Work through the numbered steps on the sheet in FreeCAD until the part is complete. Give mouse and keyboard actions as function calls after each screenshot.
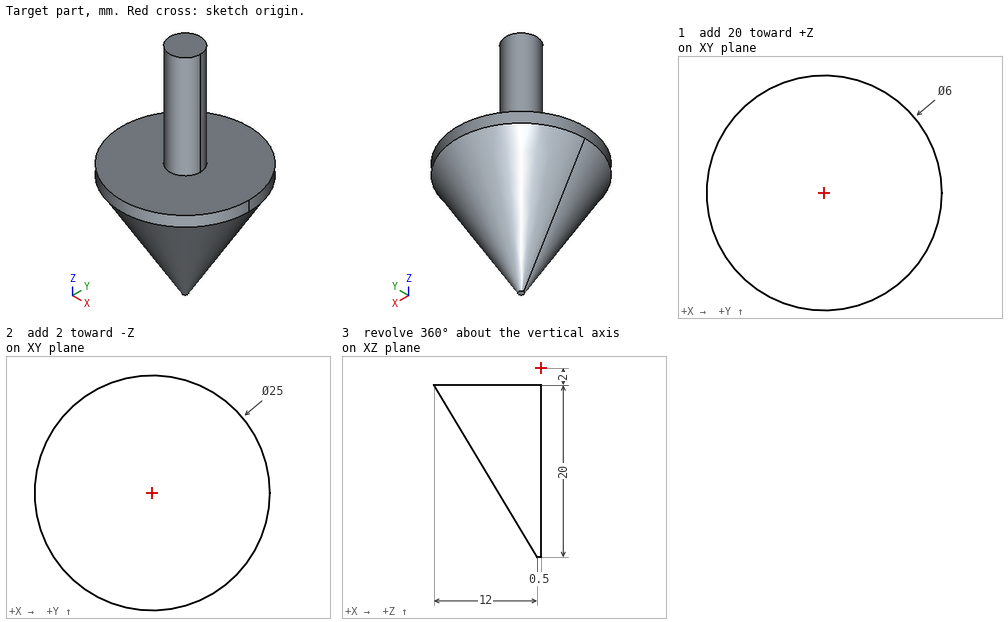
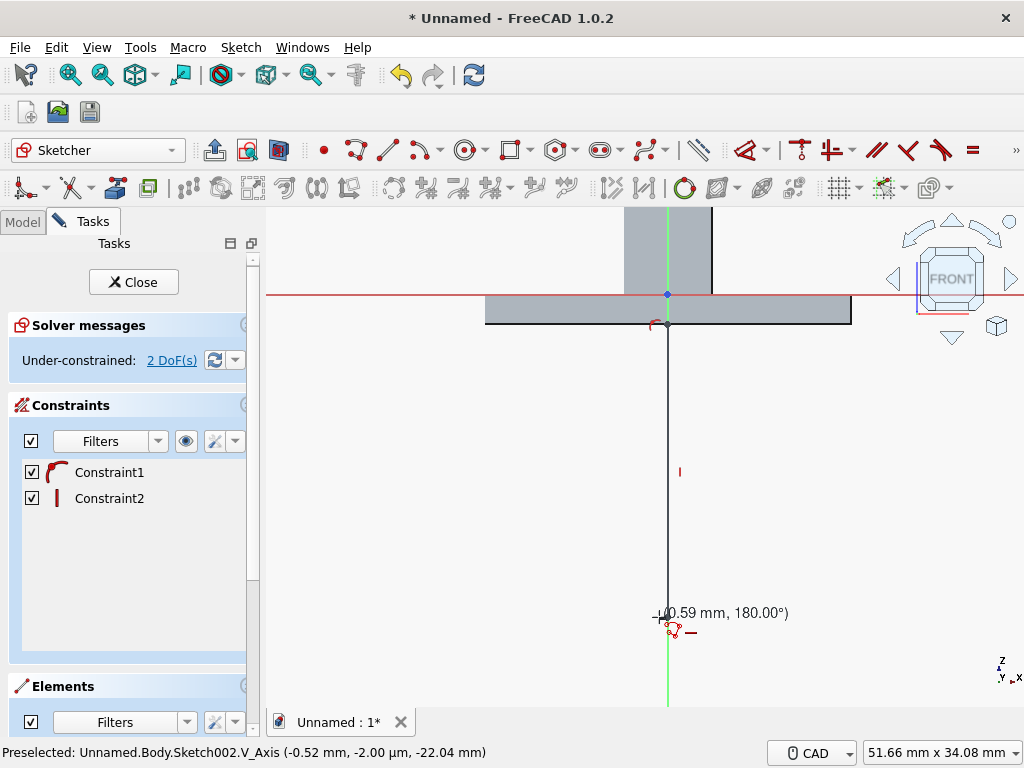
scroll(660, 617, up, 4)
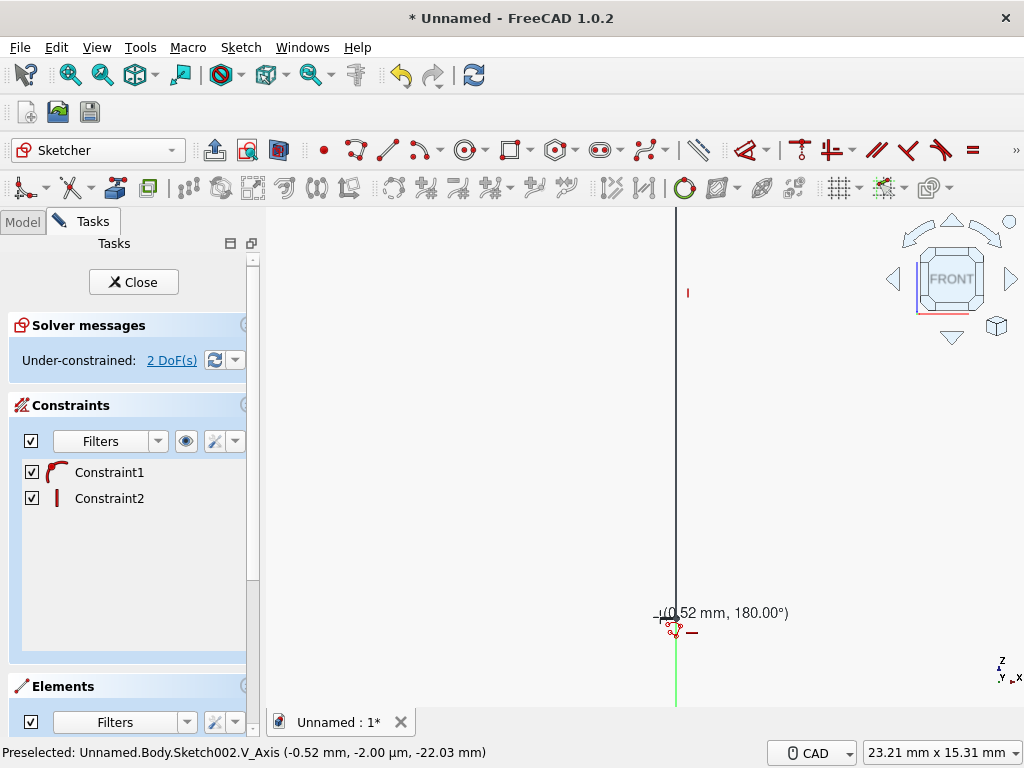
click(660, 616)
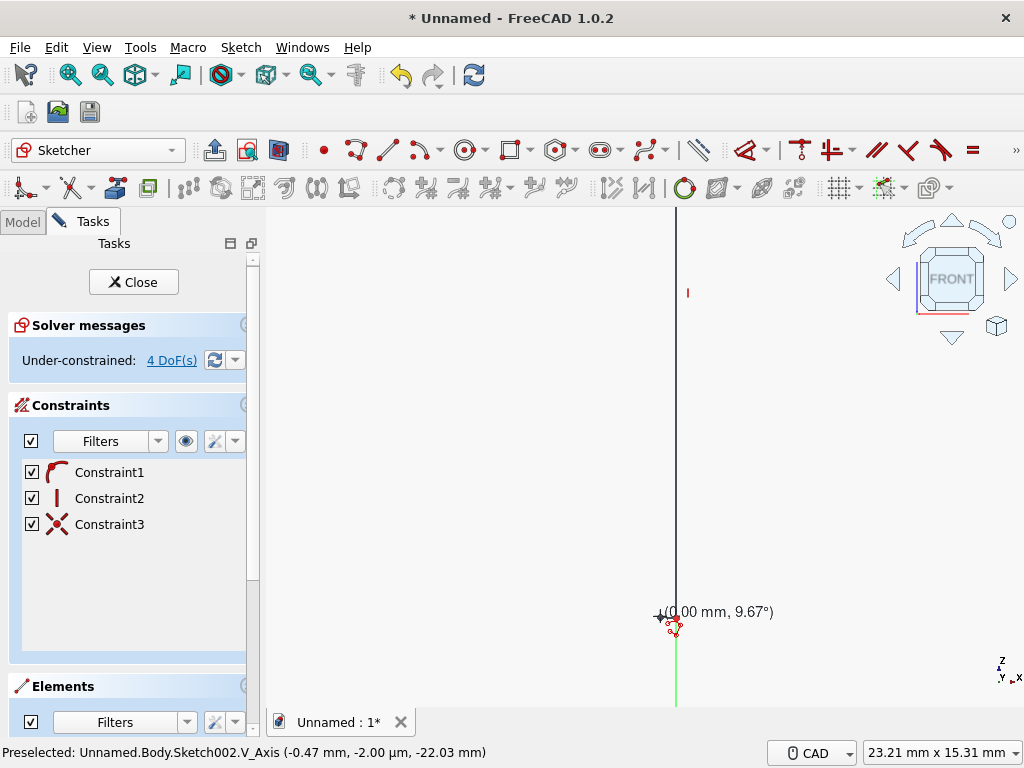
scroll(662, 619, down, 4)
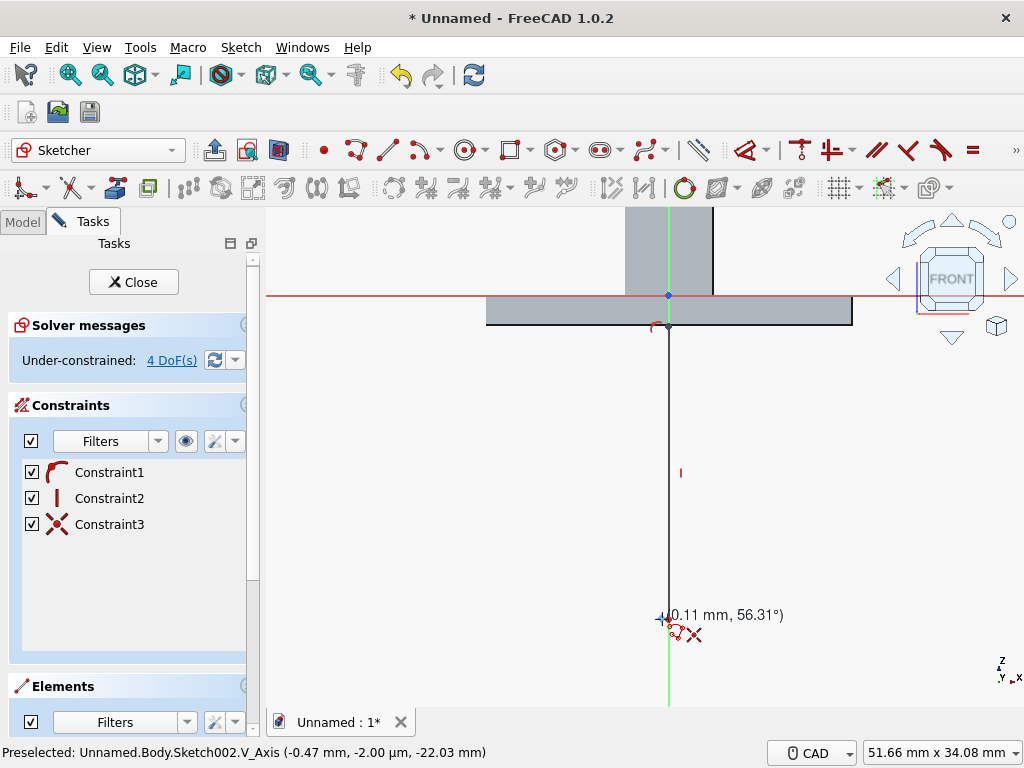
click(485, 325)
click(669, 326)
key(Escape)
key(Escape)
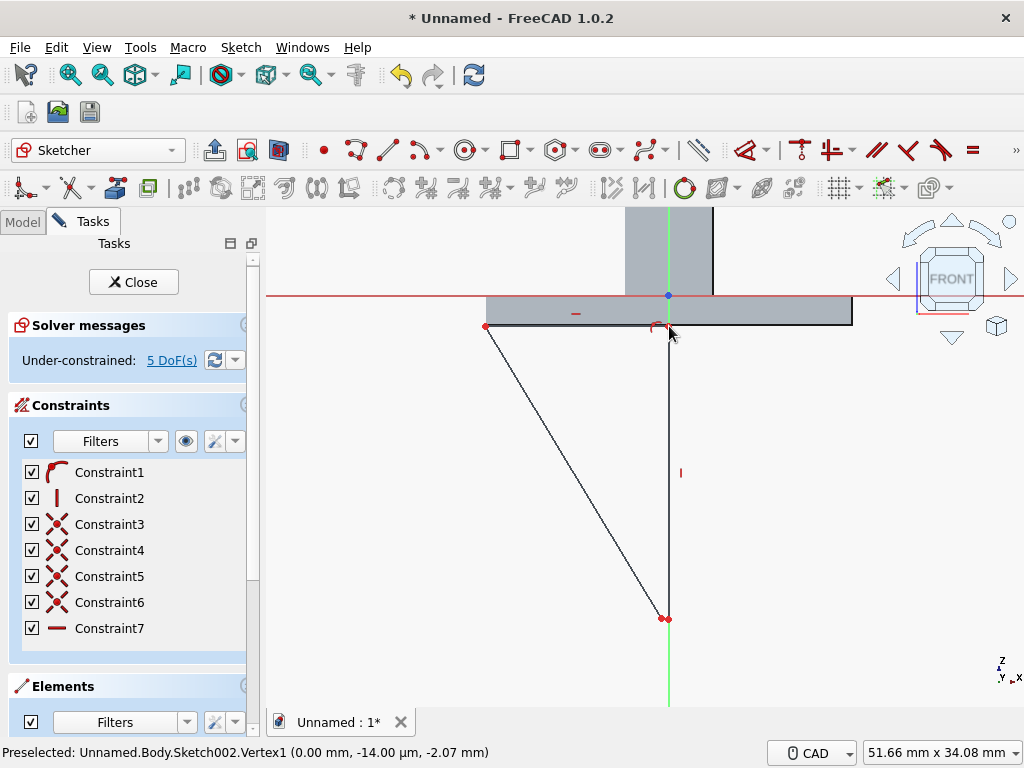
scroll(665, 619, up, 7)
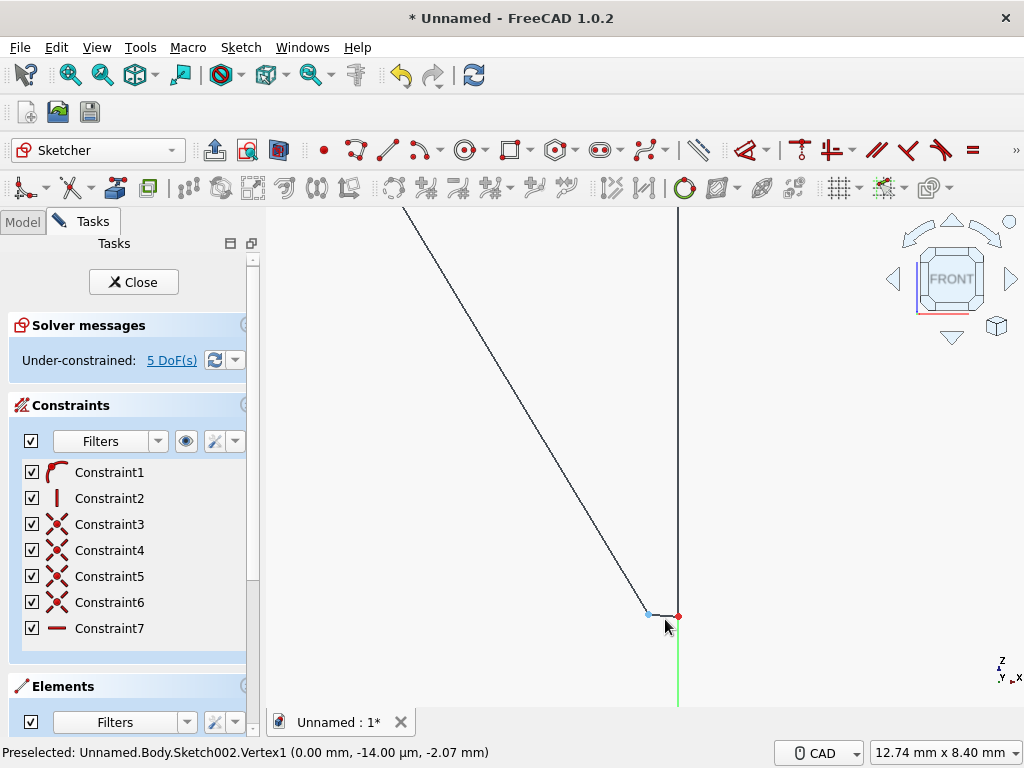
click(664, 616)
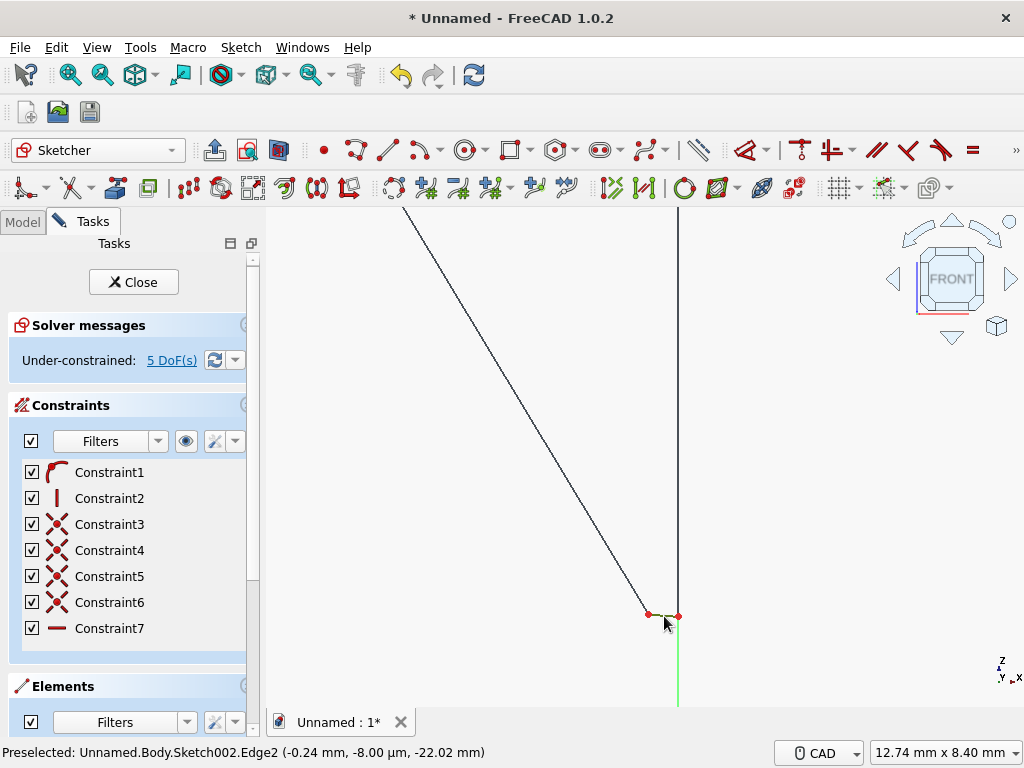
key(h)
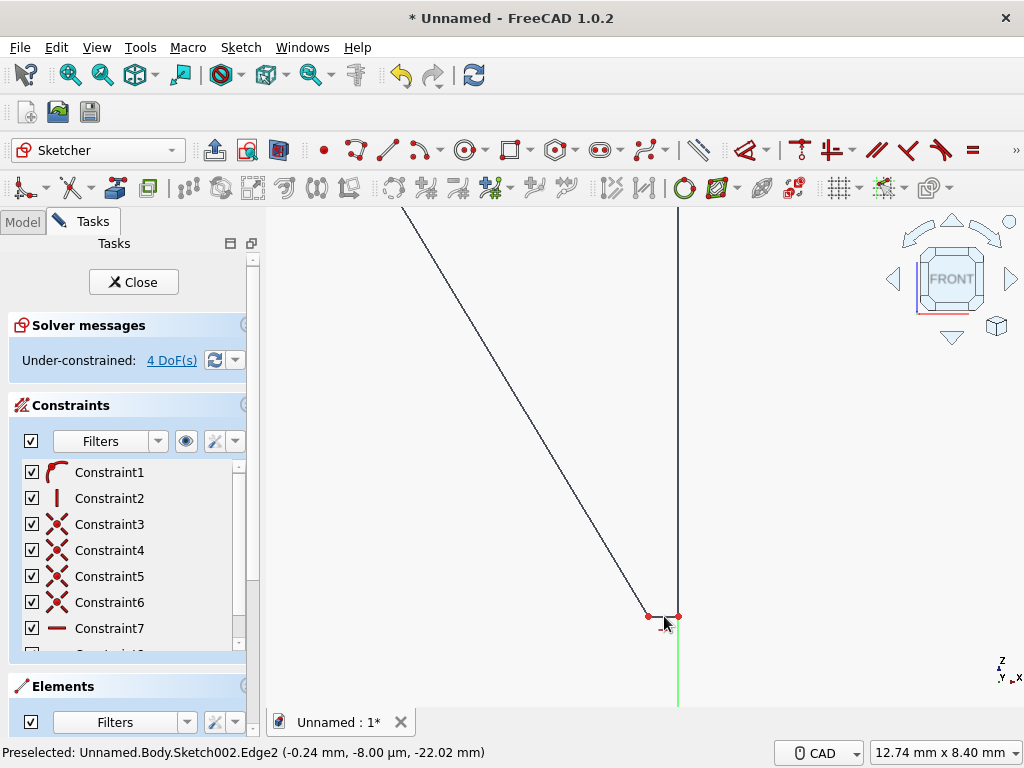
click(746, 150)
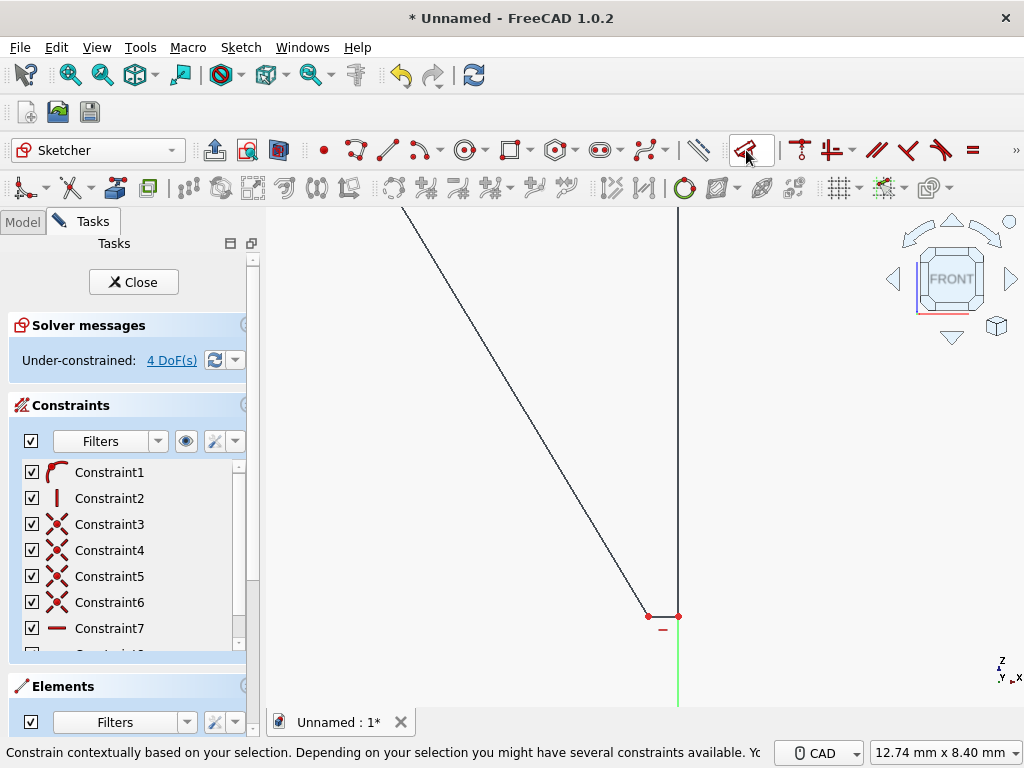
scroll(665, 620, down, 7)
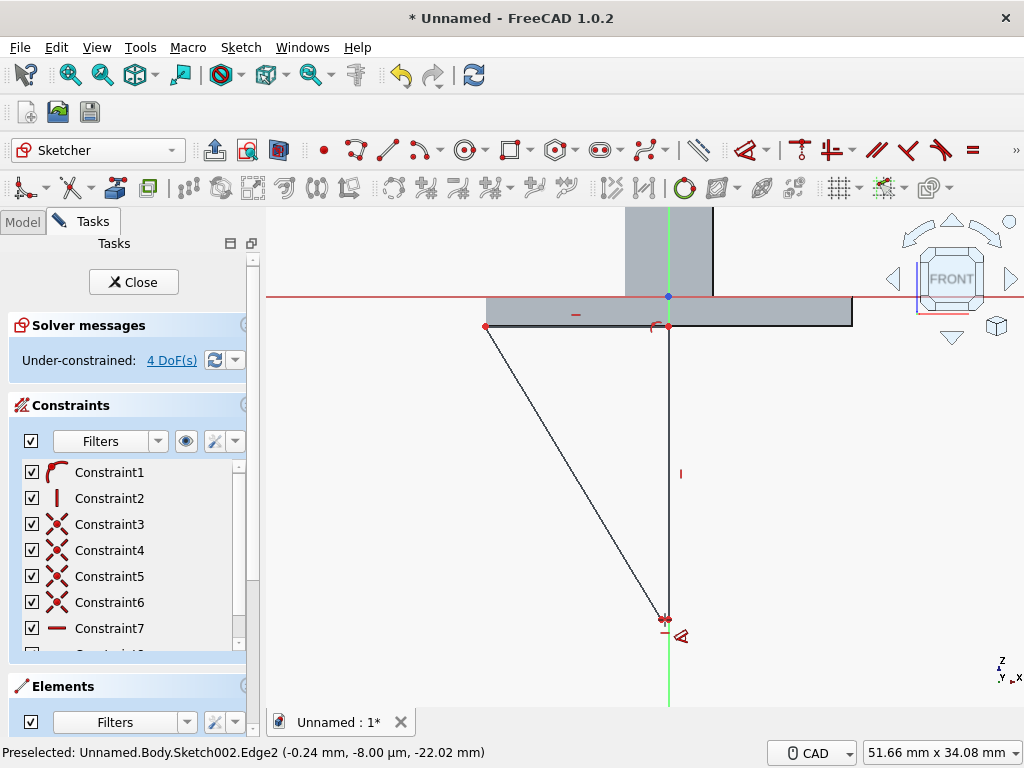
click(669, 532)
click(703, 473)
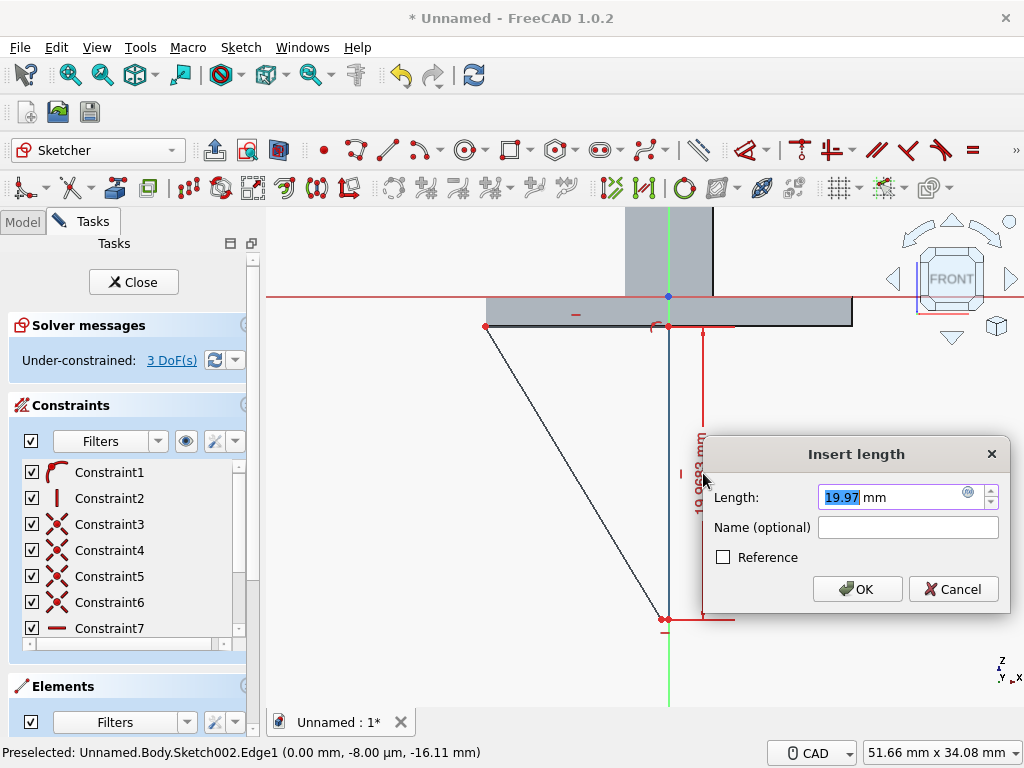
text(20)
key(Return)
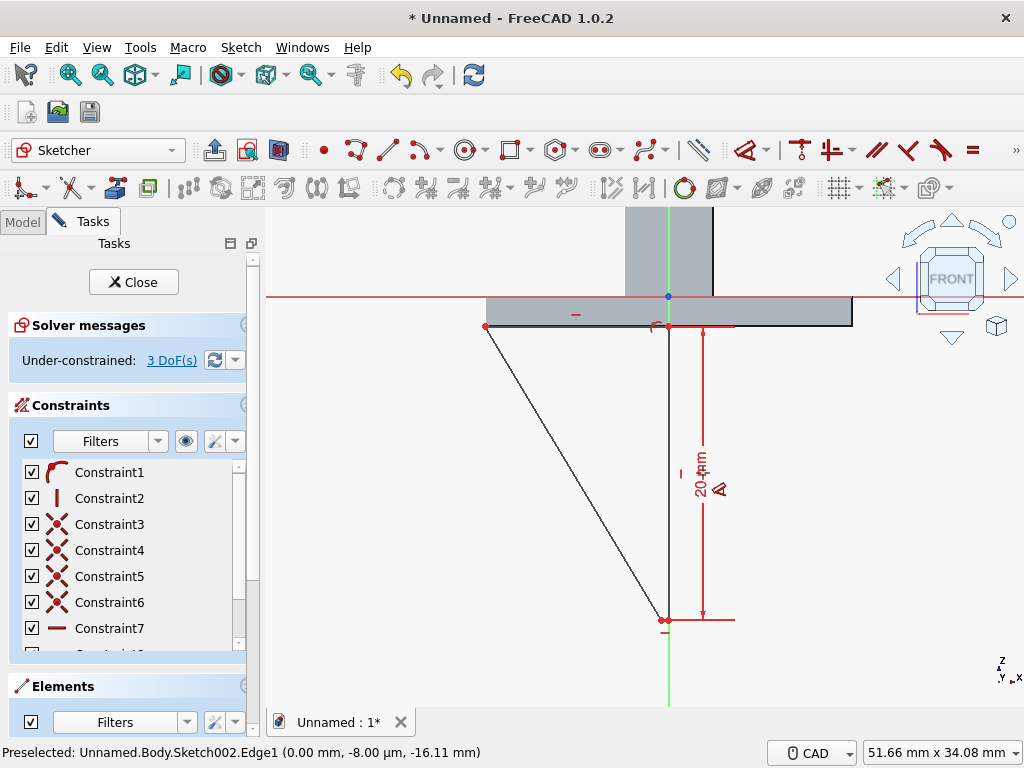
scroll(669, 327, up, 2)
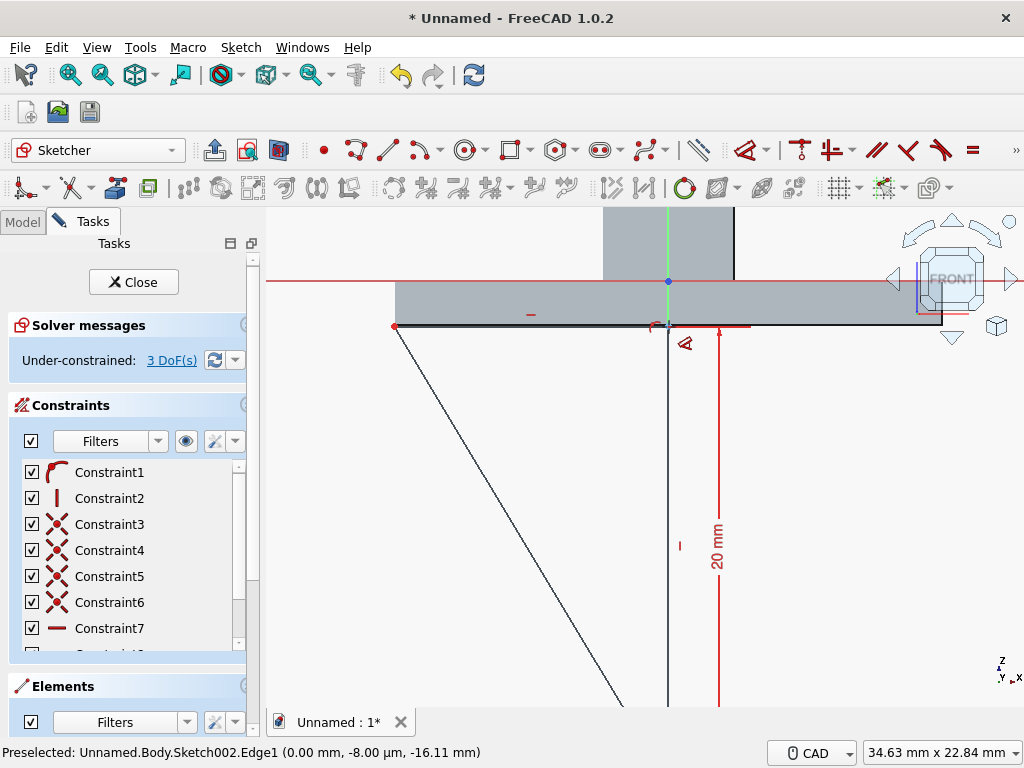
click(668, 327)
click(702, 304)